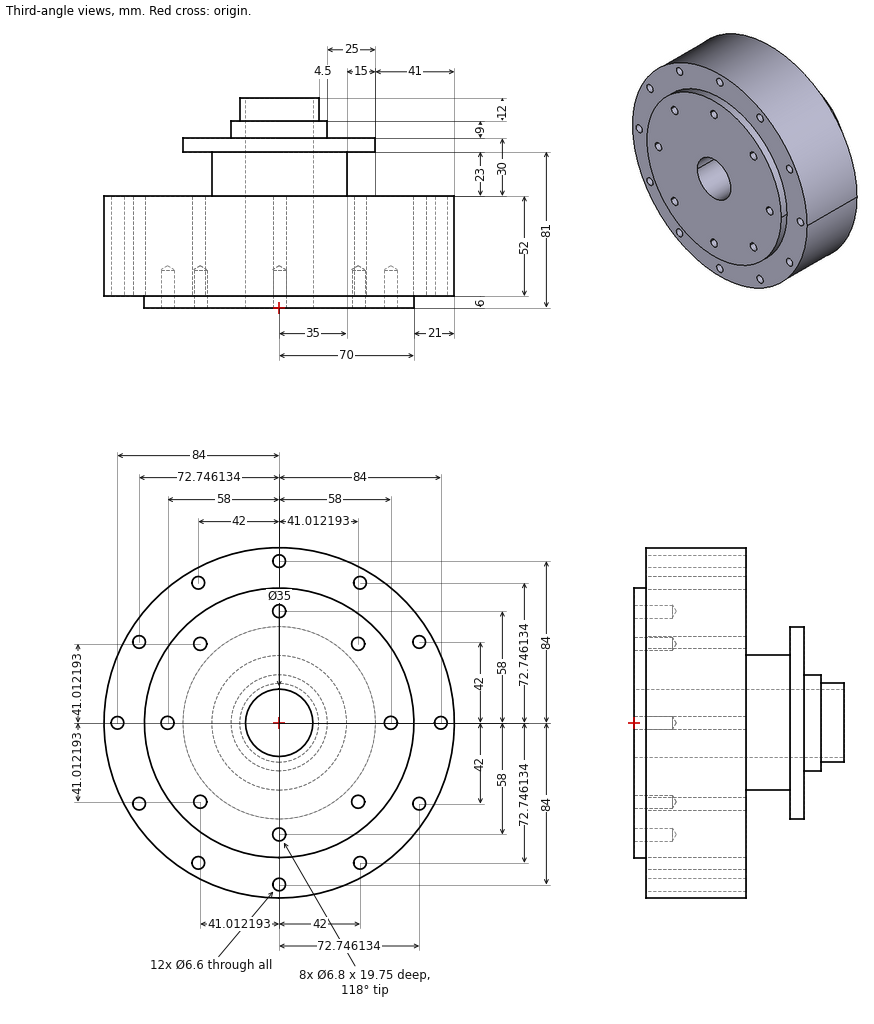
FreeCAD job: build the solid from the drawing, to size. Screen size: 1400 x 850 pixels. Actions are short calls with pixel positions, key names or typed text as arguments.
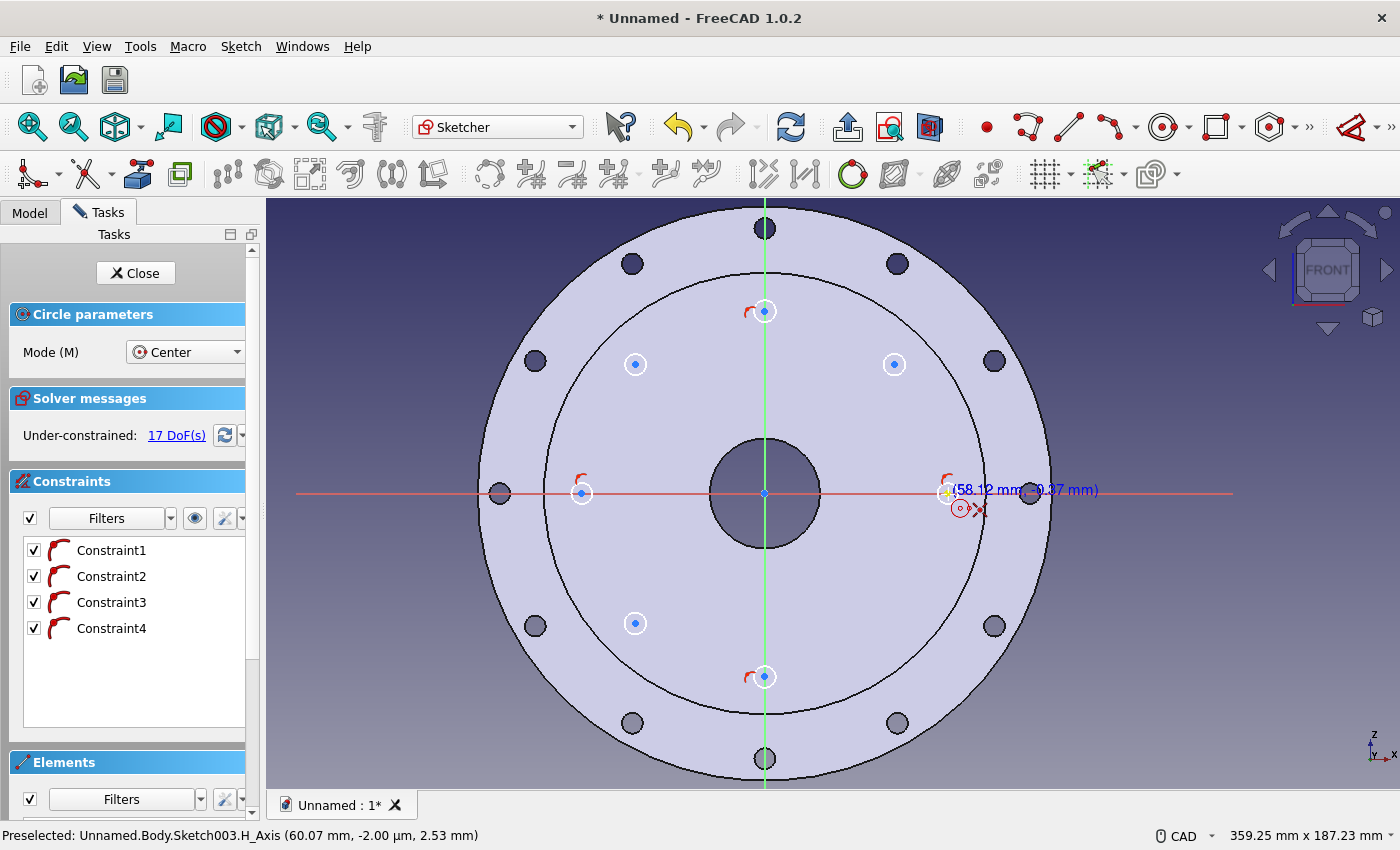
scroll(894, 623, up, 4)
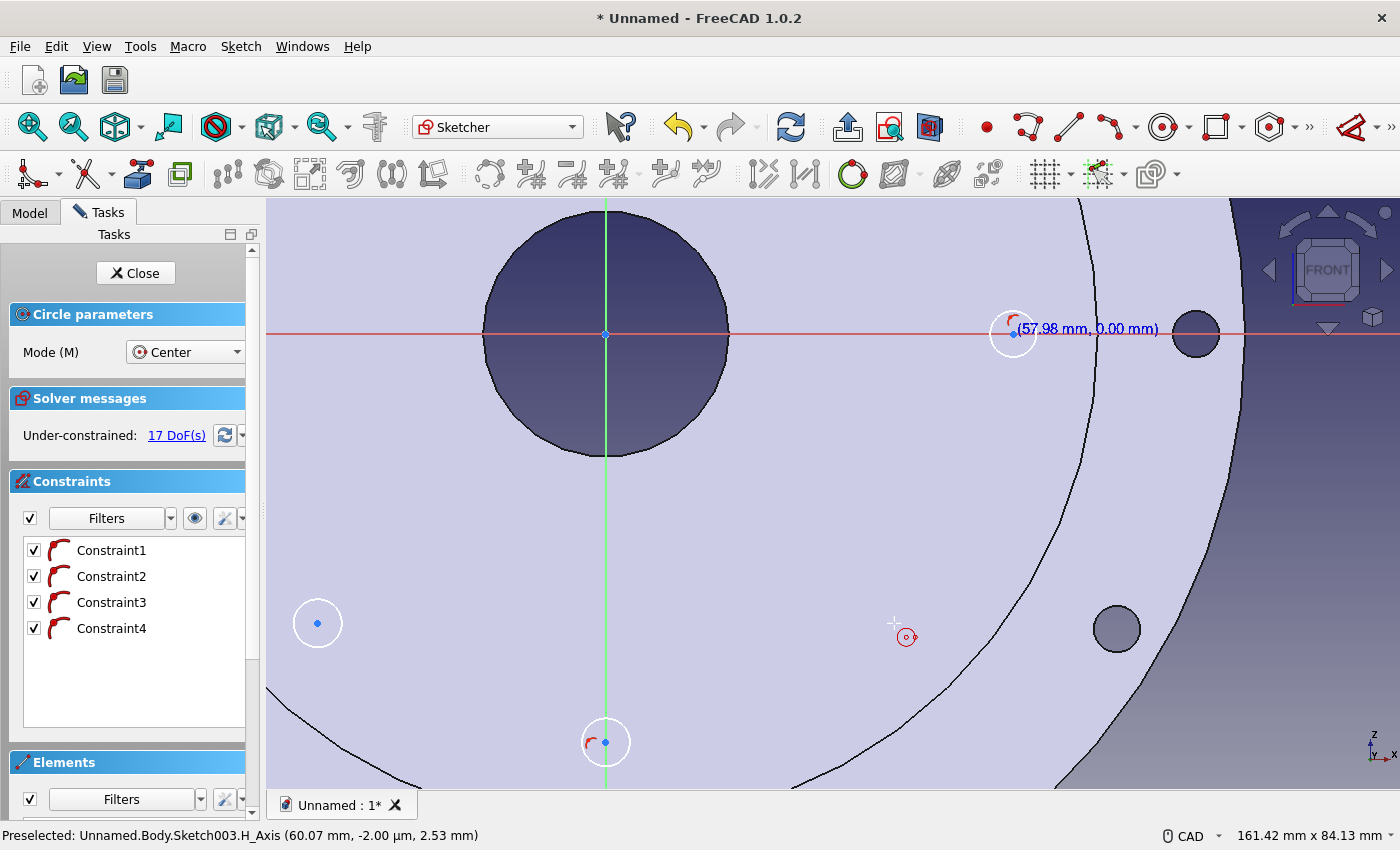
click(894, 622)
click(911, 605)
key(Escape)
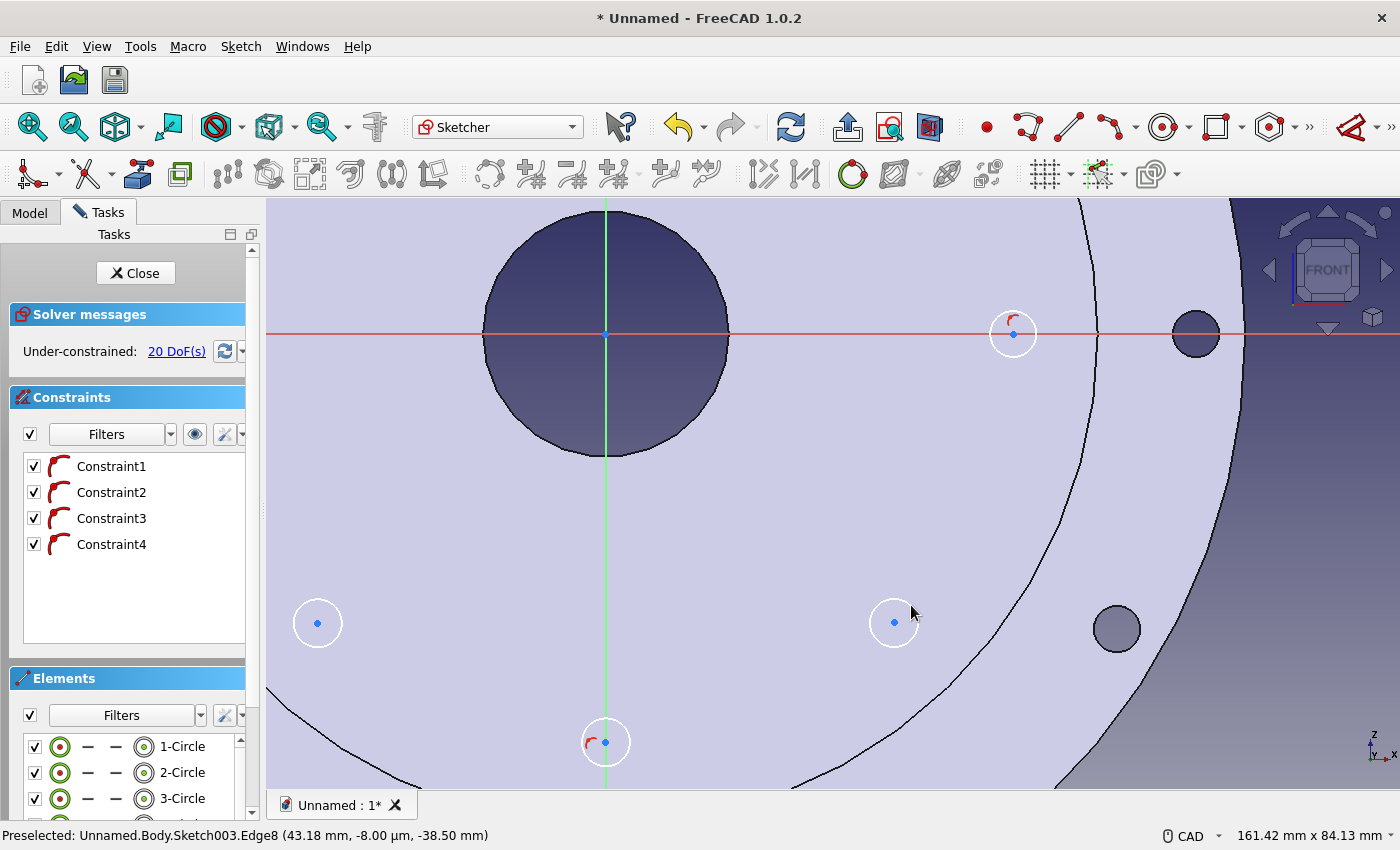
click(623, 725)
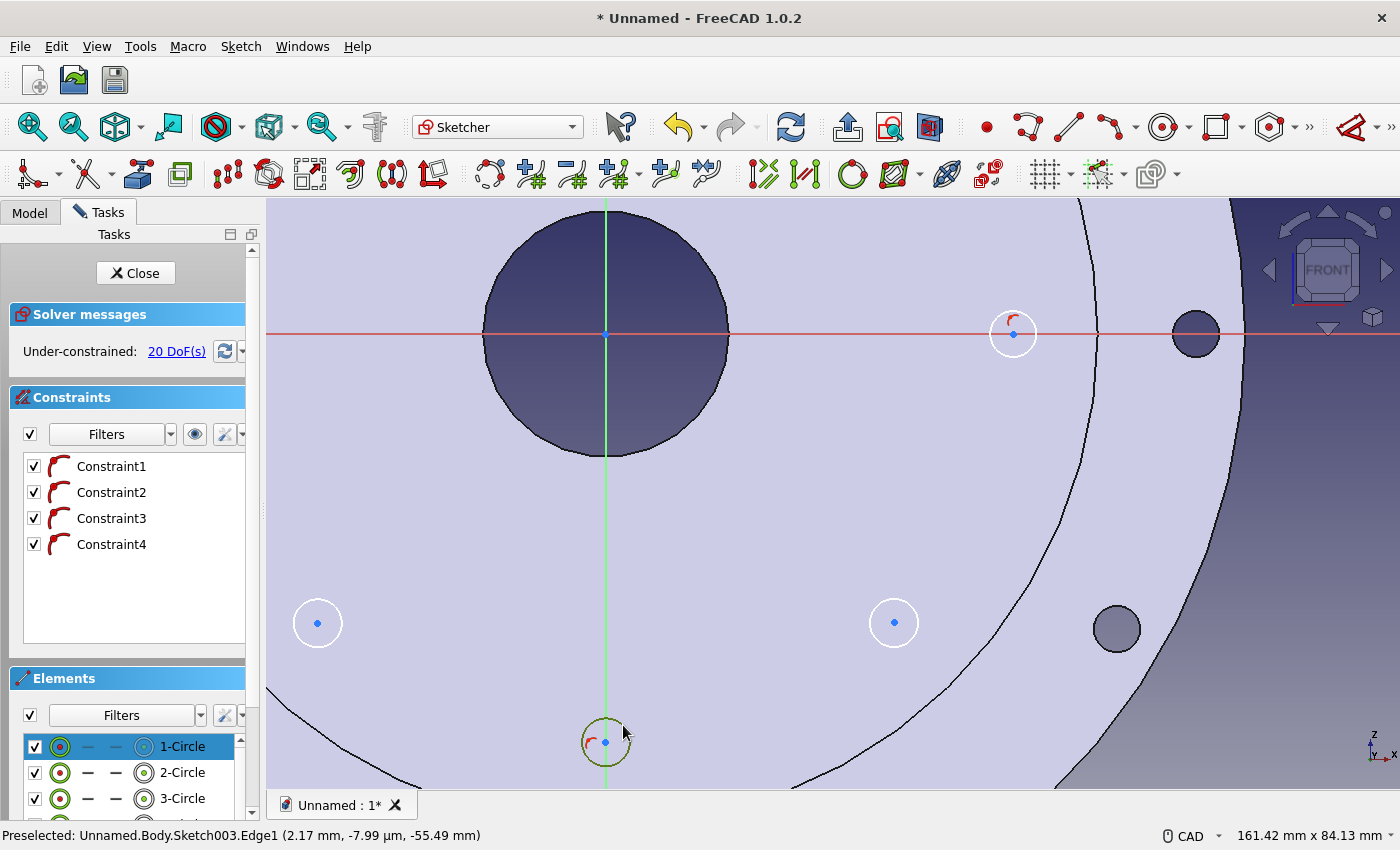
click(335, 606)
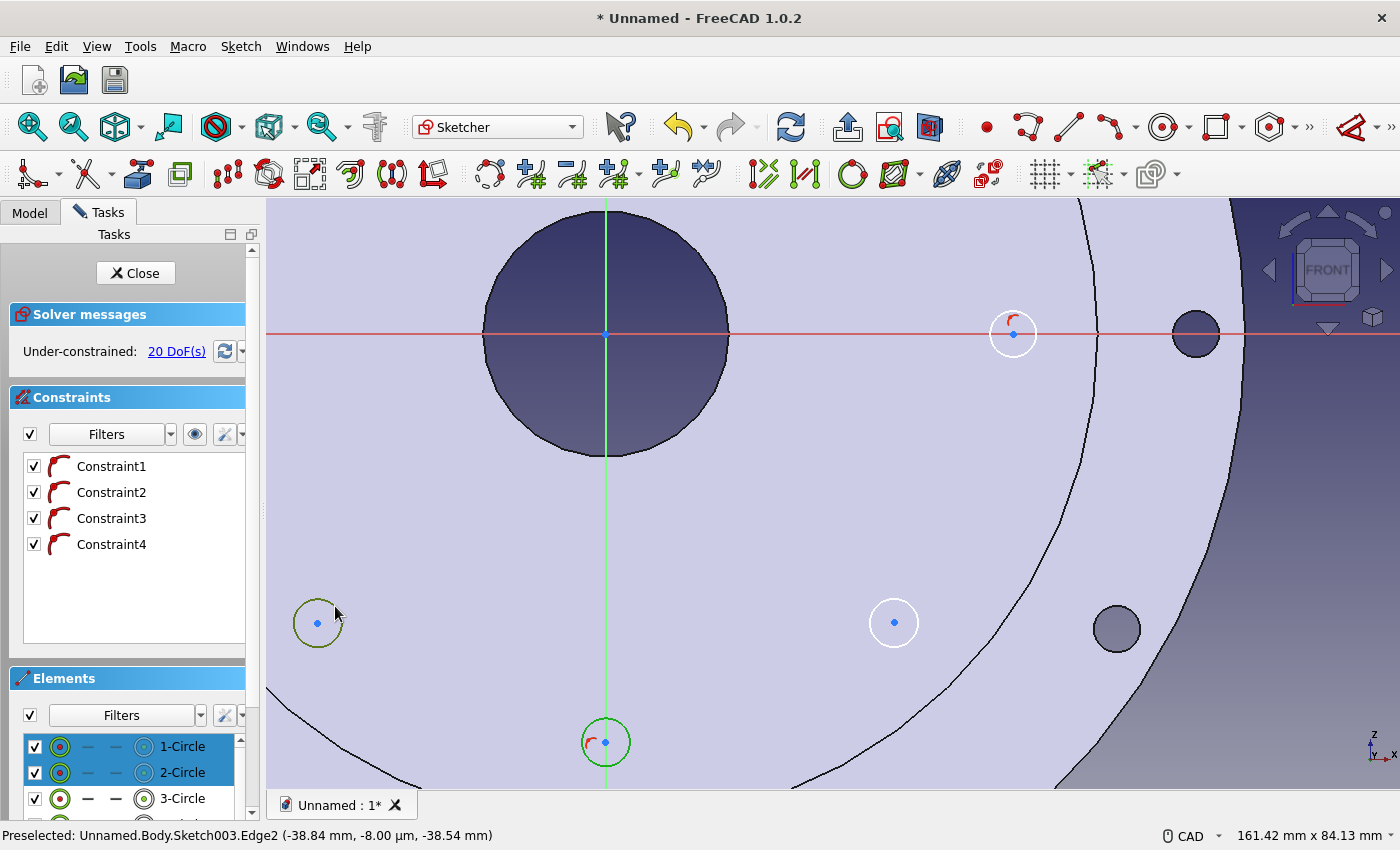
scroll(894, 624, down, 4)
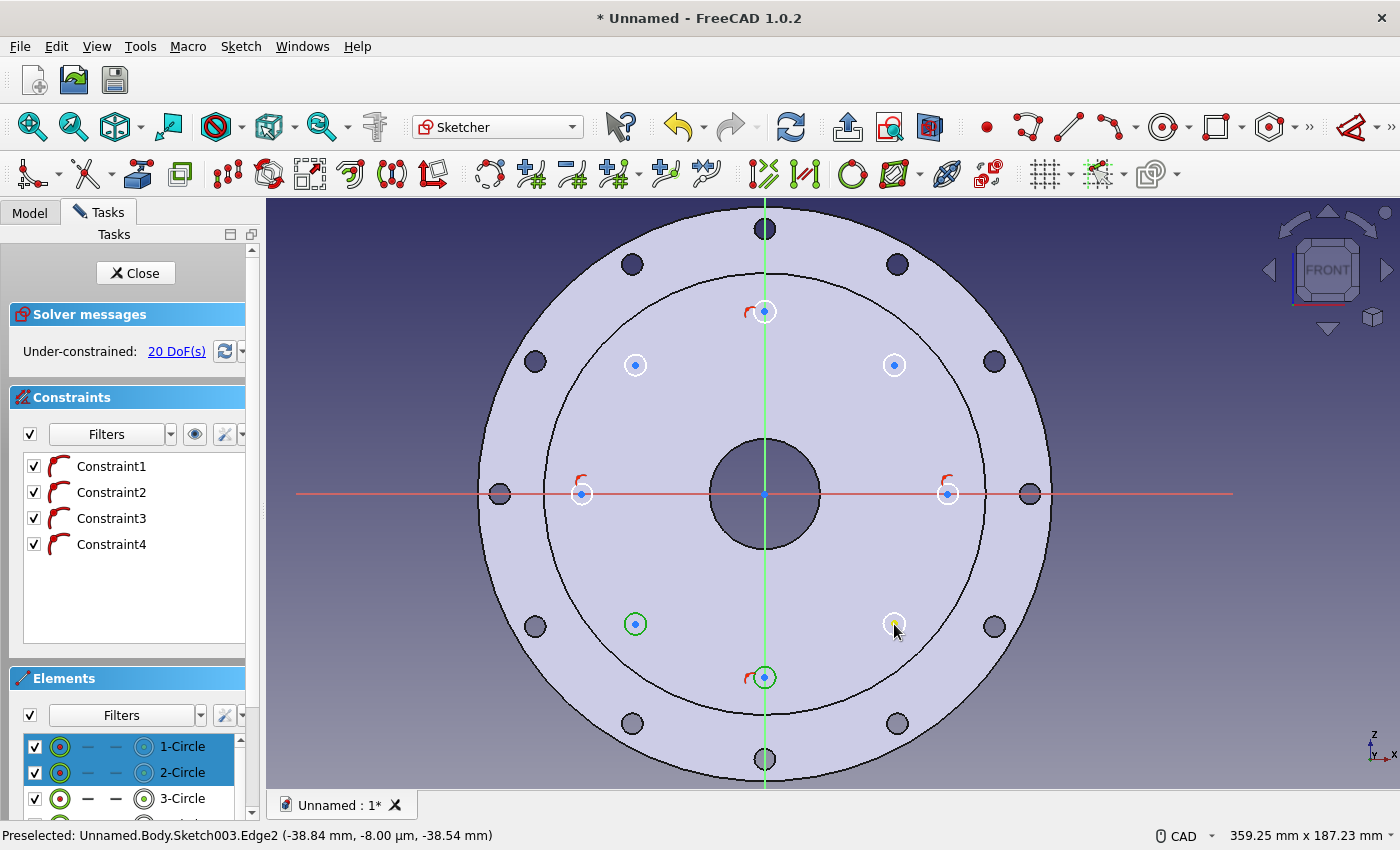
scroll(589, 487, up, 4)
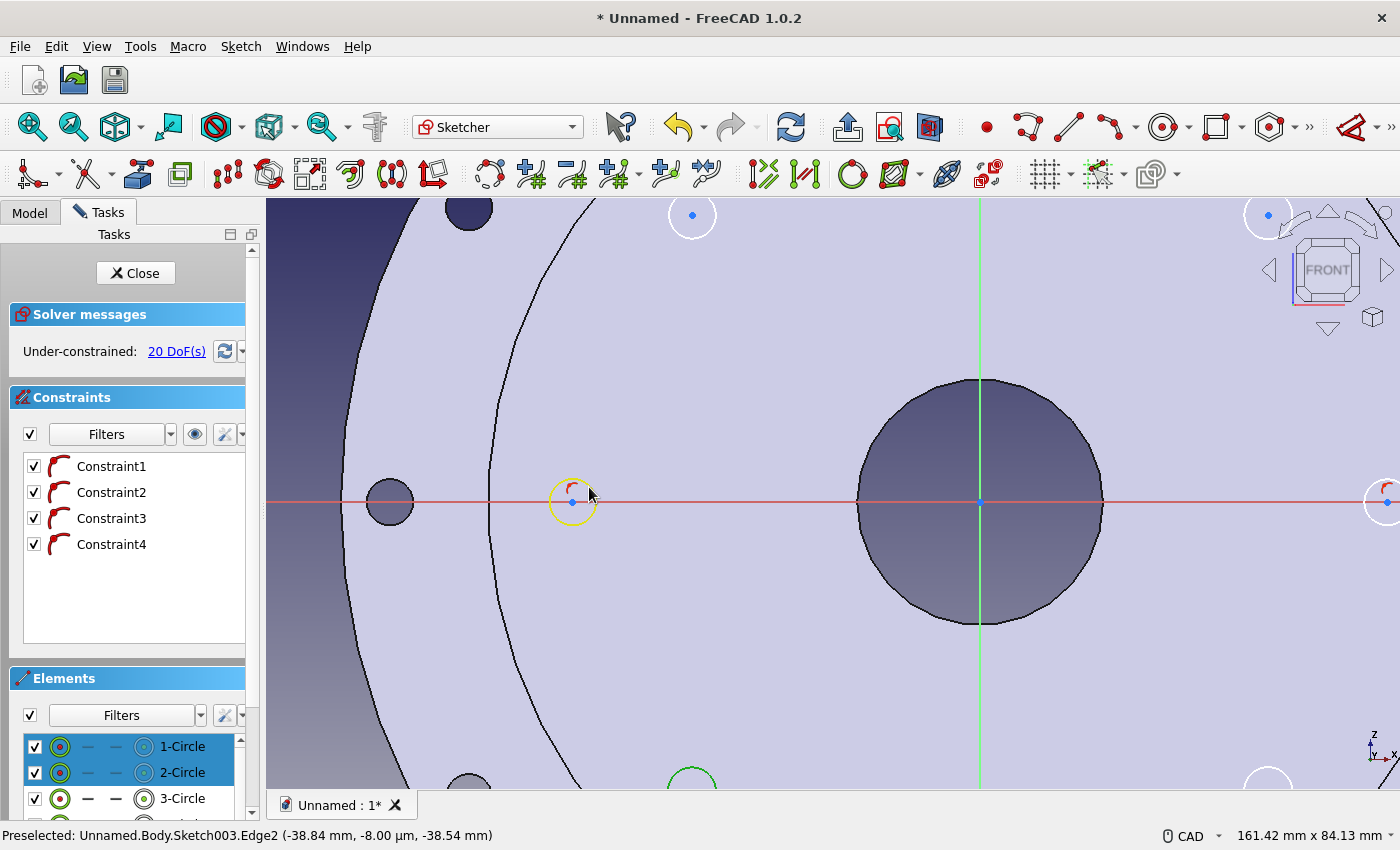
click(589, 486)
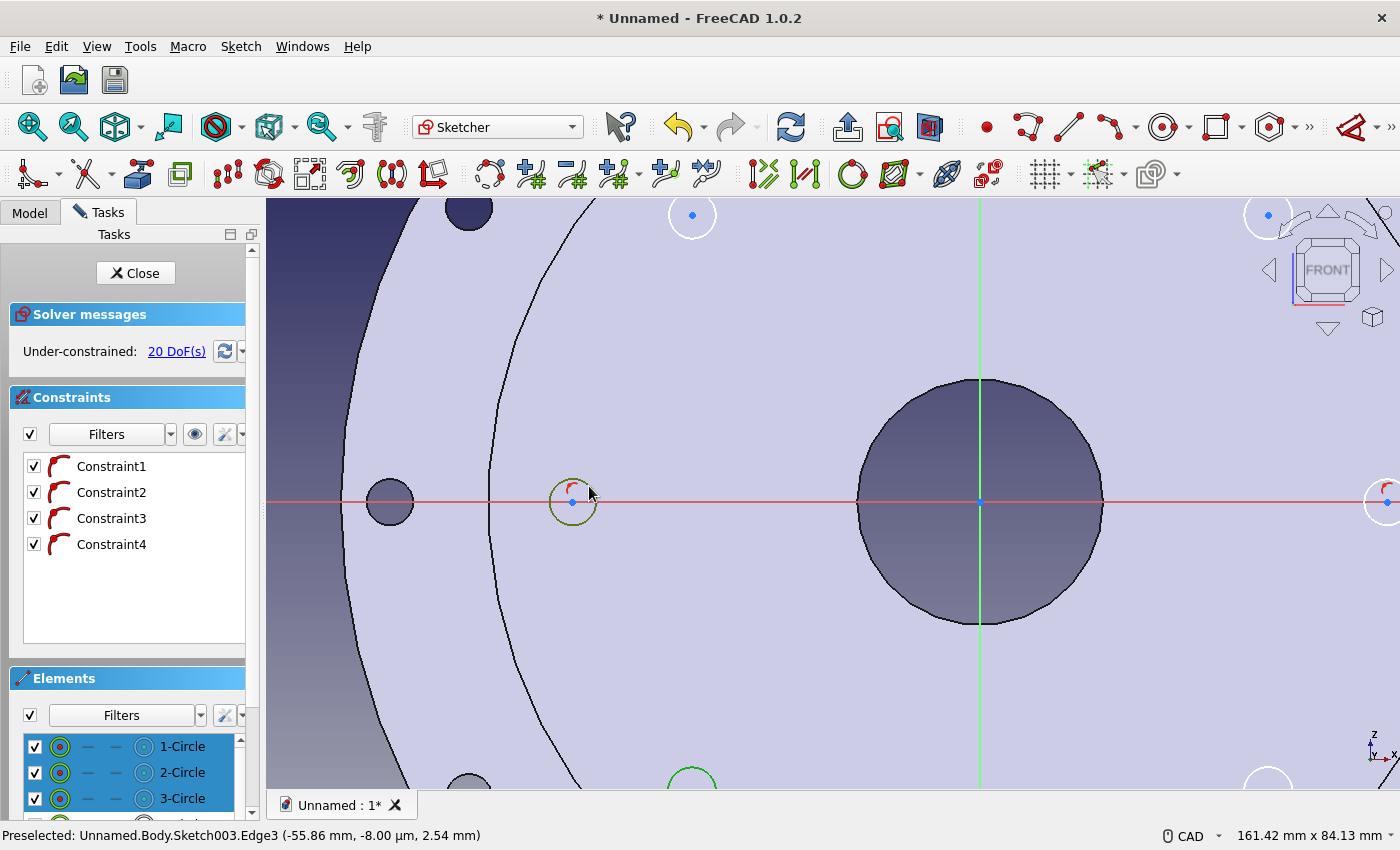
click(676, 232)